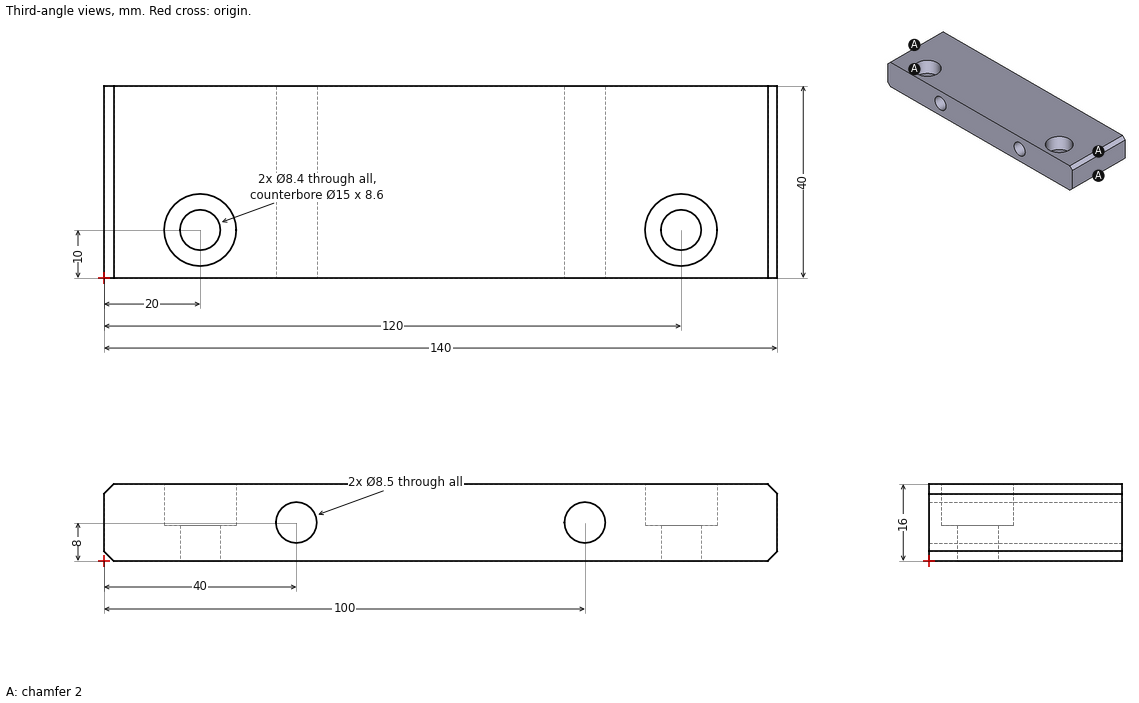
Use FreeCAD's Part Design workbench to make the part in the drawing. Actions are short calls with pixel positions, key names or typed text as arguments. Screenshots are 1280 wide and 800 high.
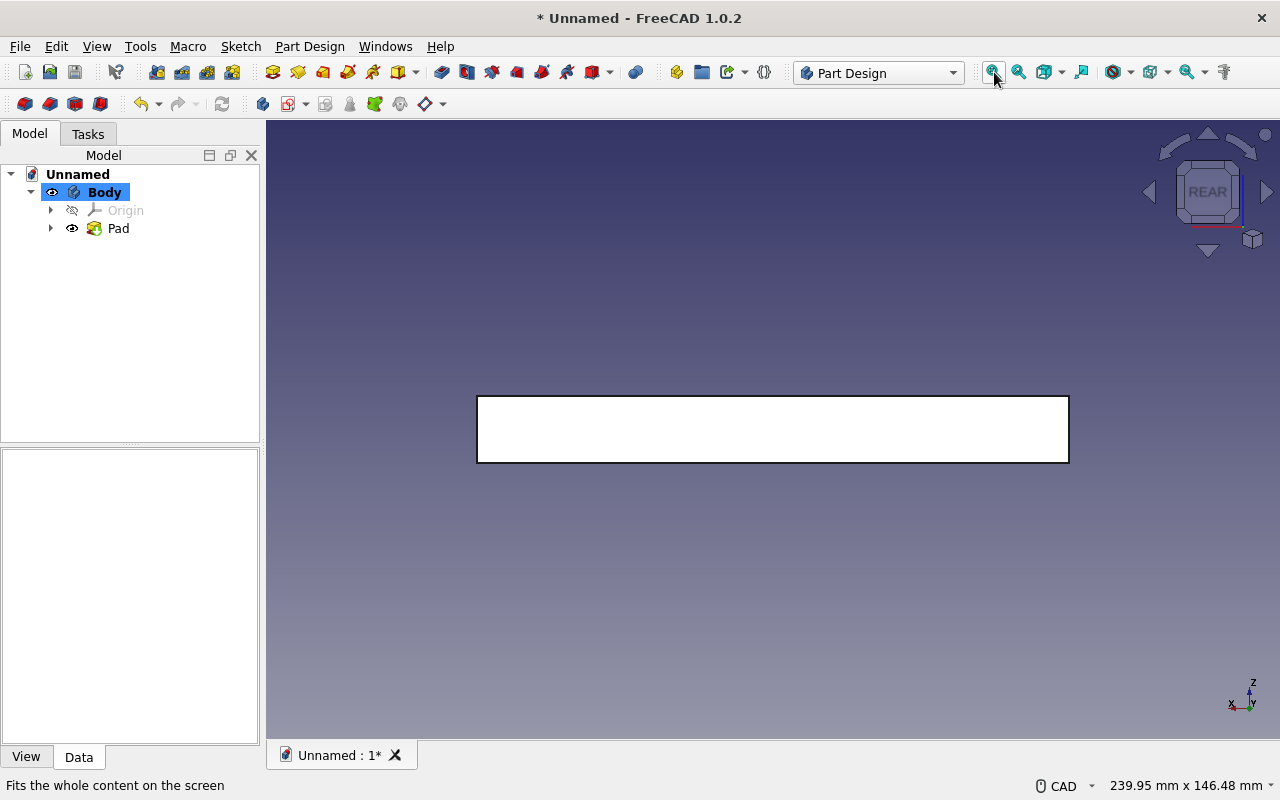
click(519, 428)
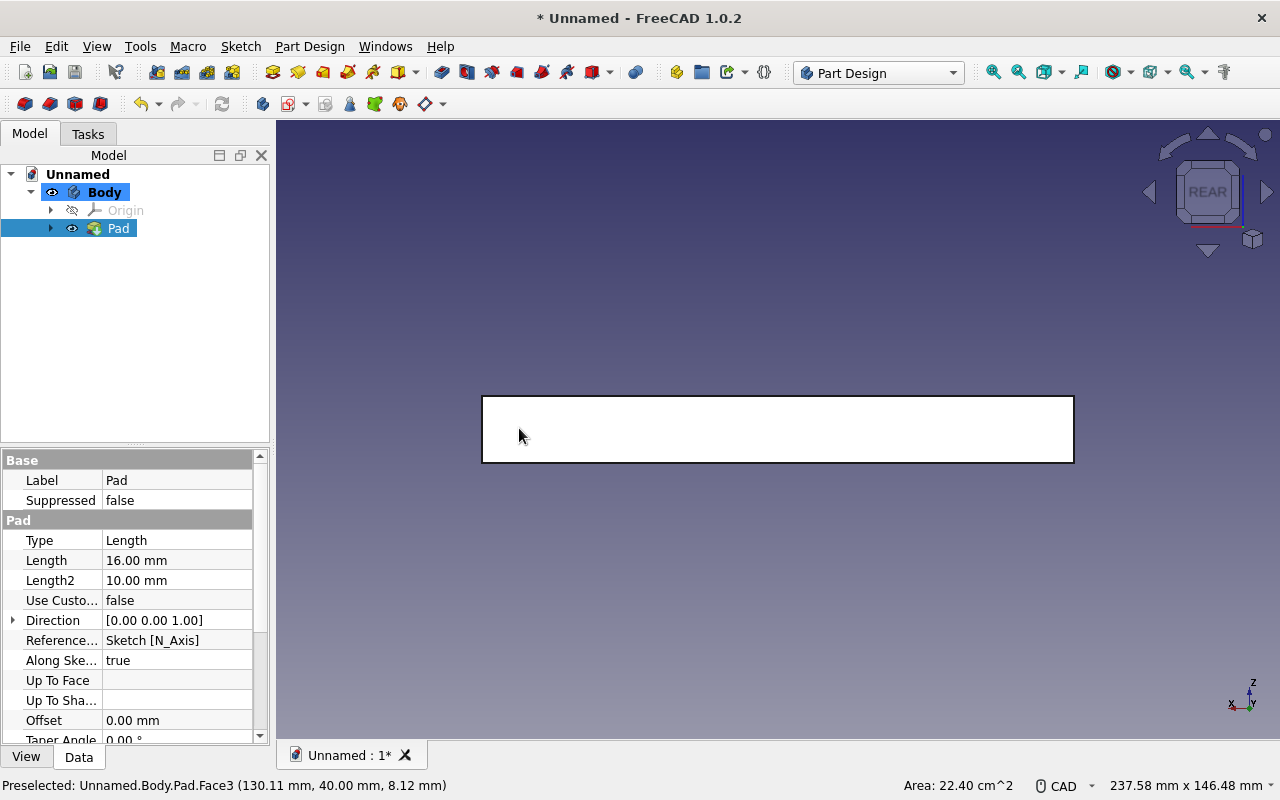
click(288, 104)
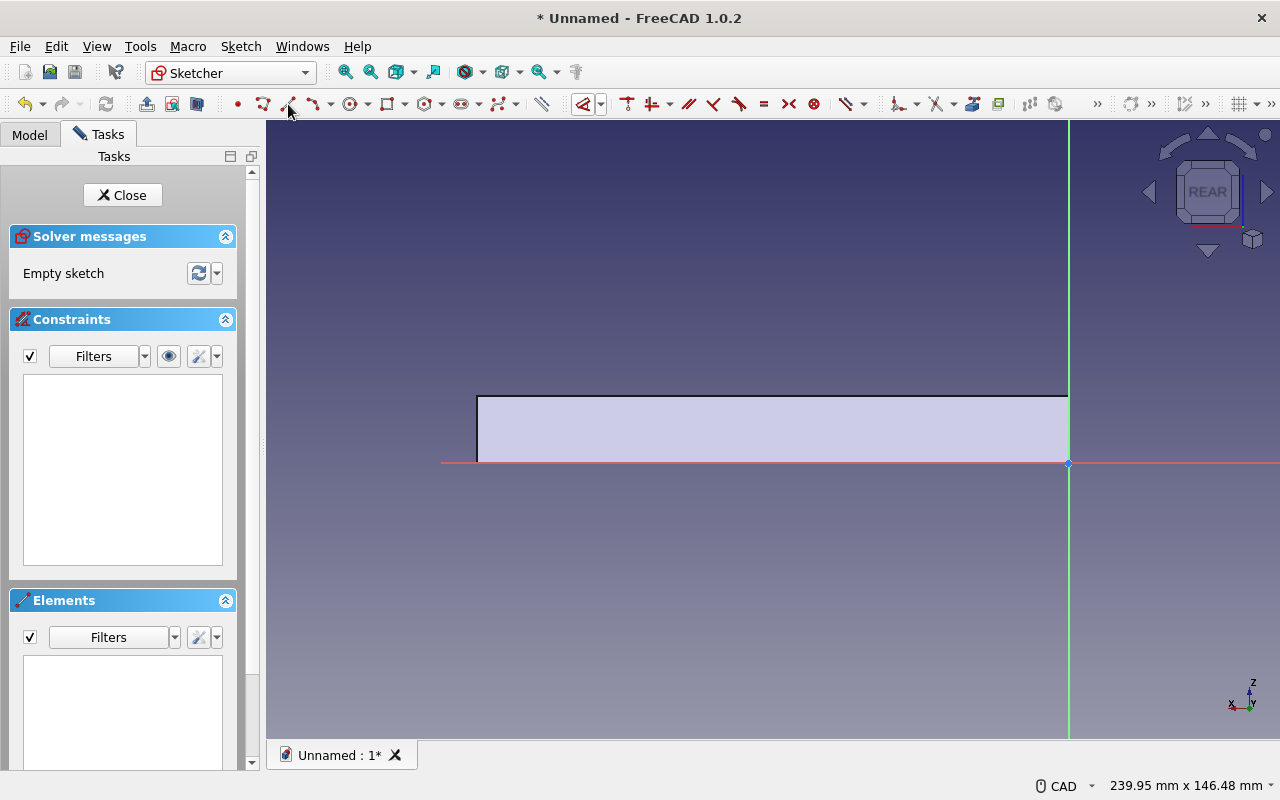
click(350, 104)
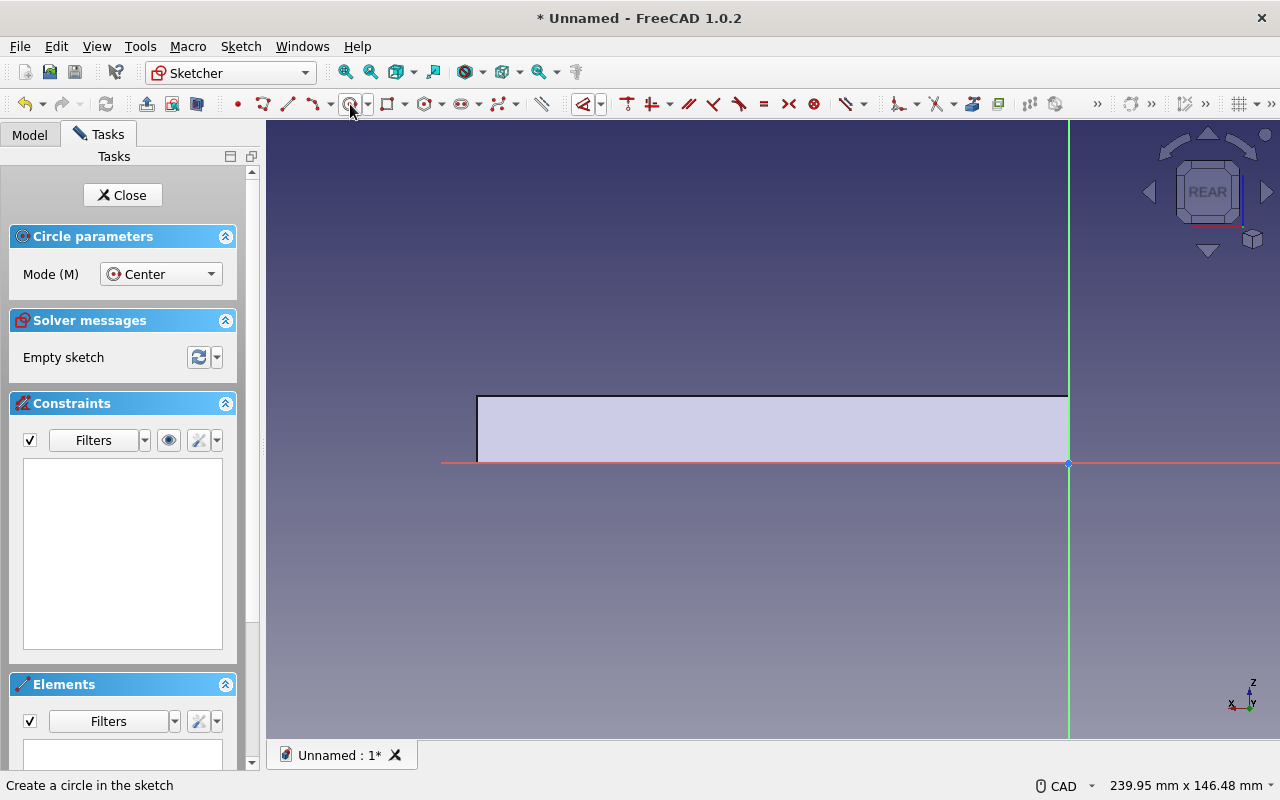
scroll(900, 429, up, 2)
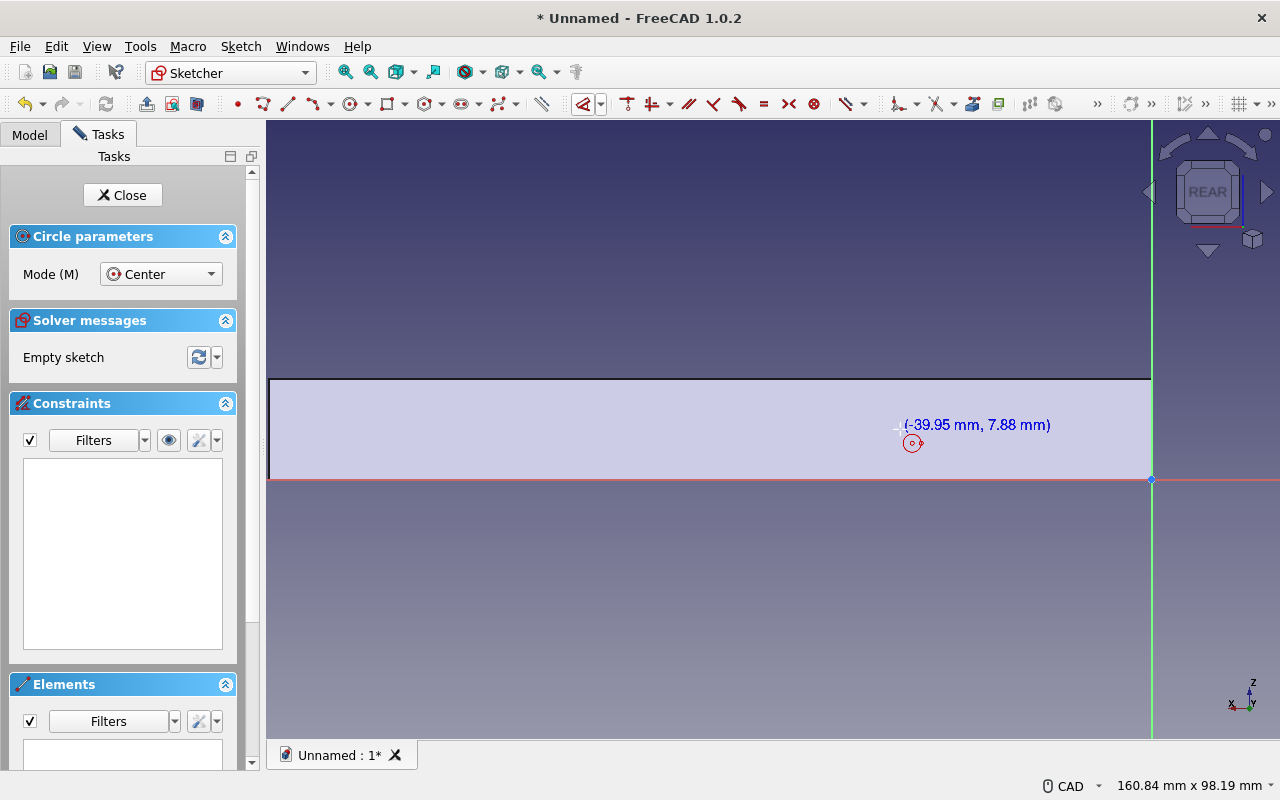
click(899, 429)
click(918, 411)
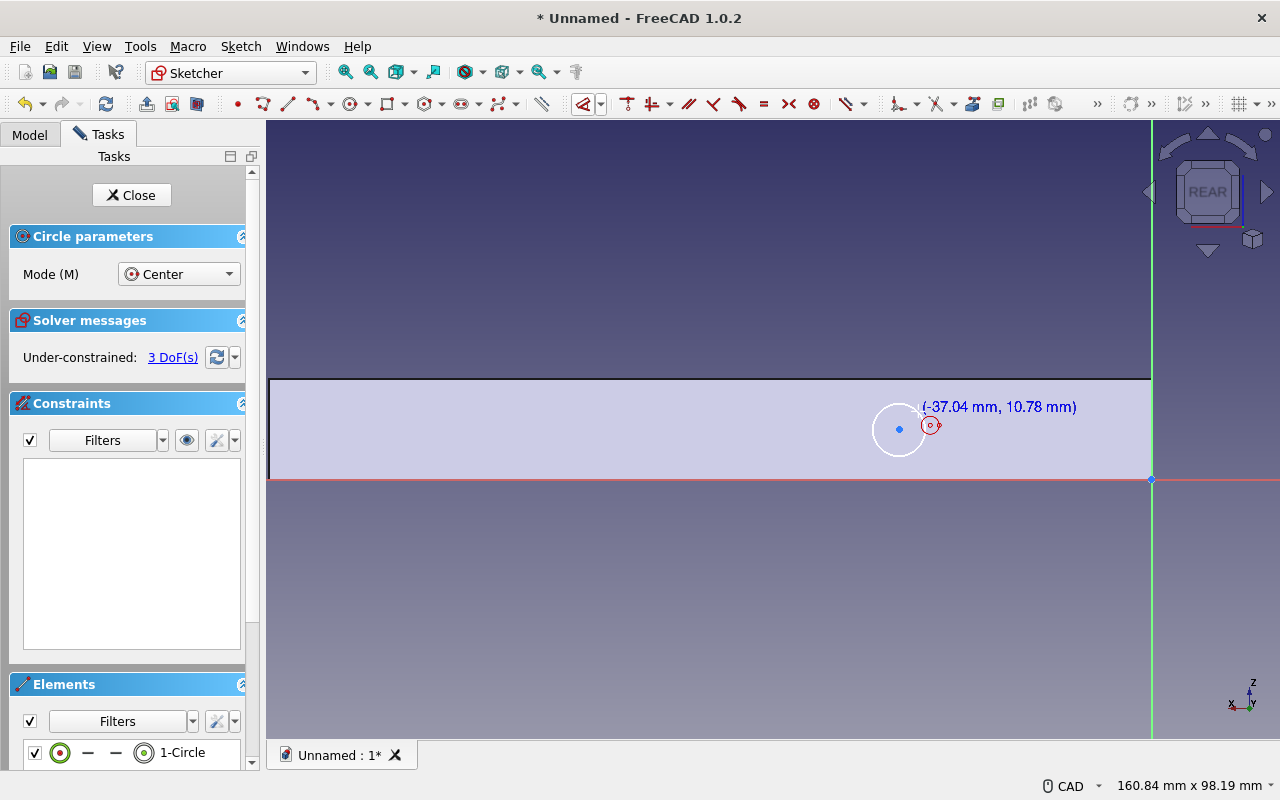
click(521, 429)
click(540, 411)
key(Escape)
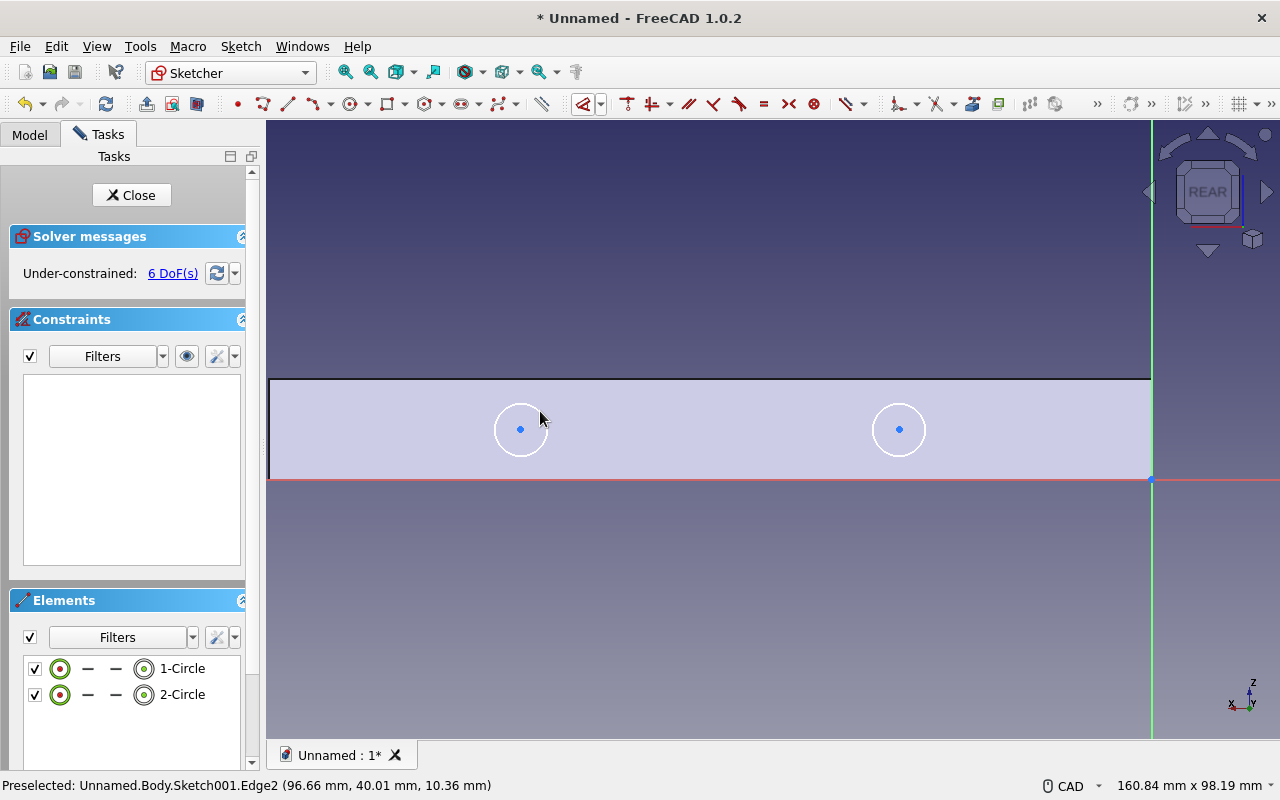
click(917, 411)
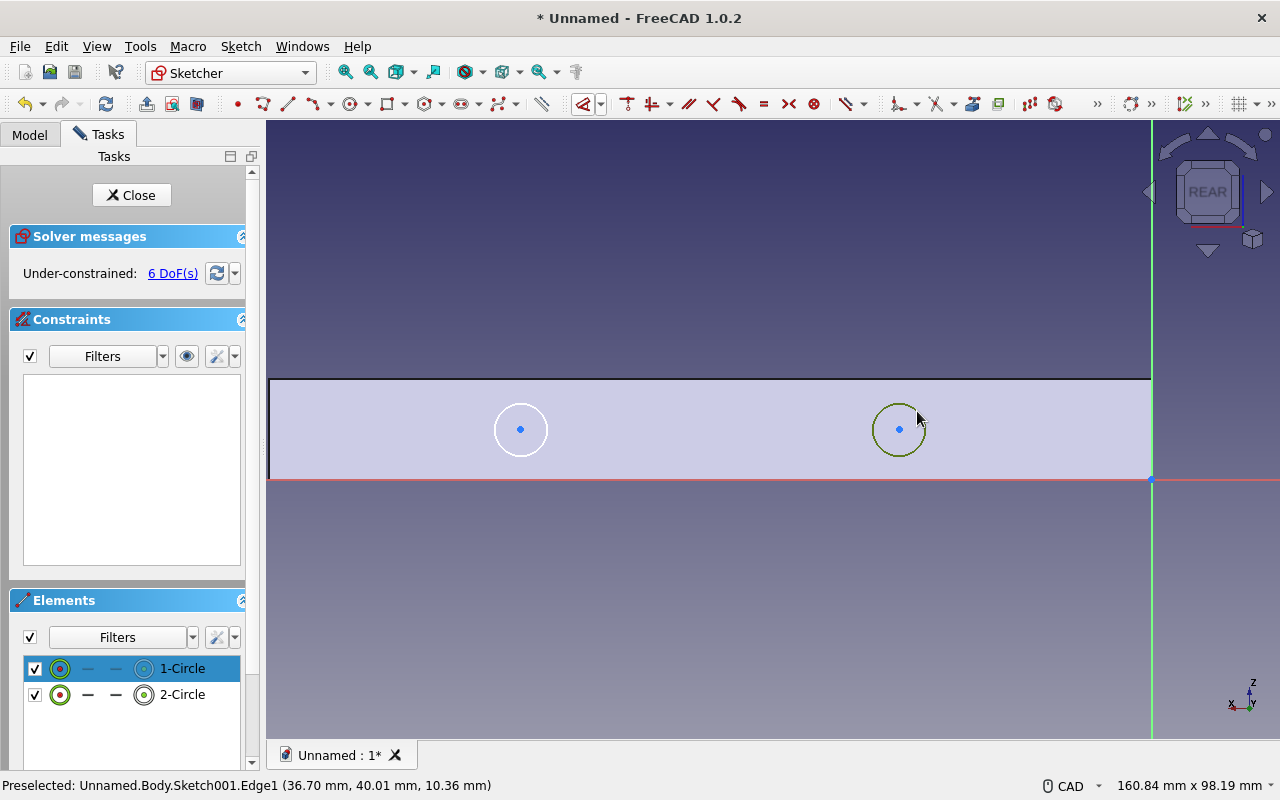
click(539, 411)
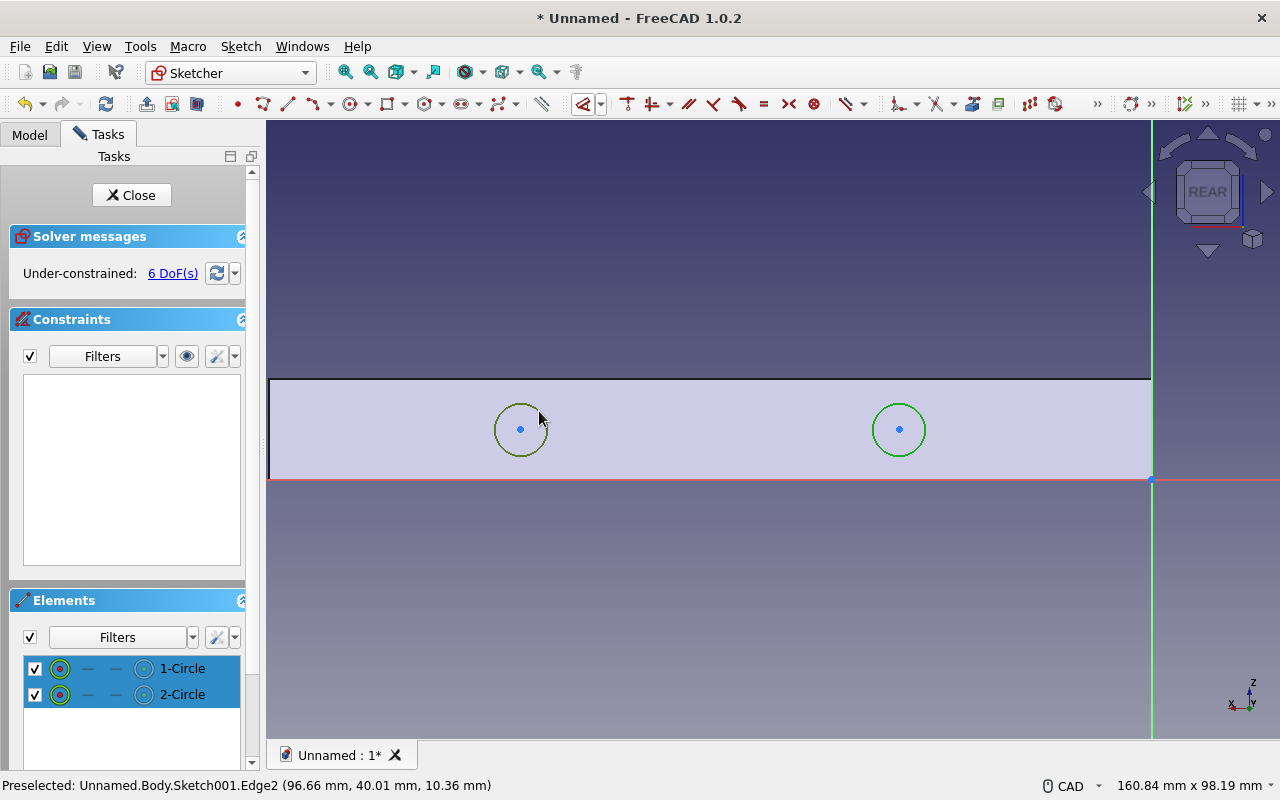
click(764, 104)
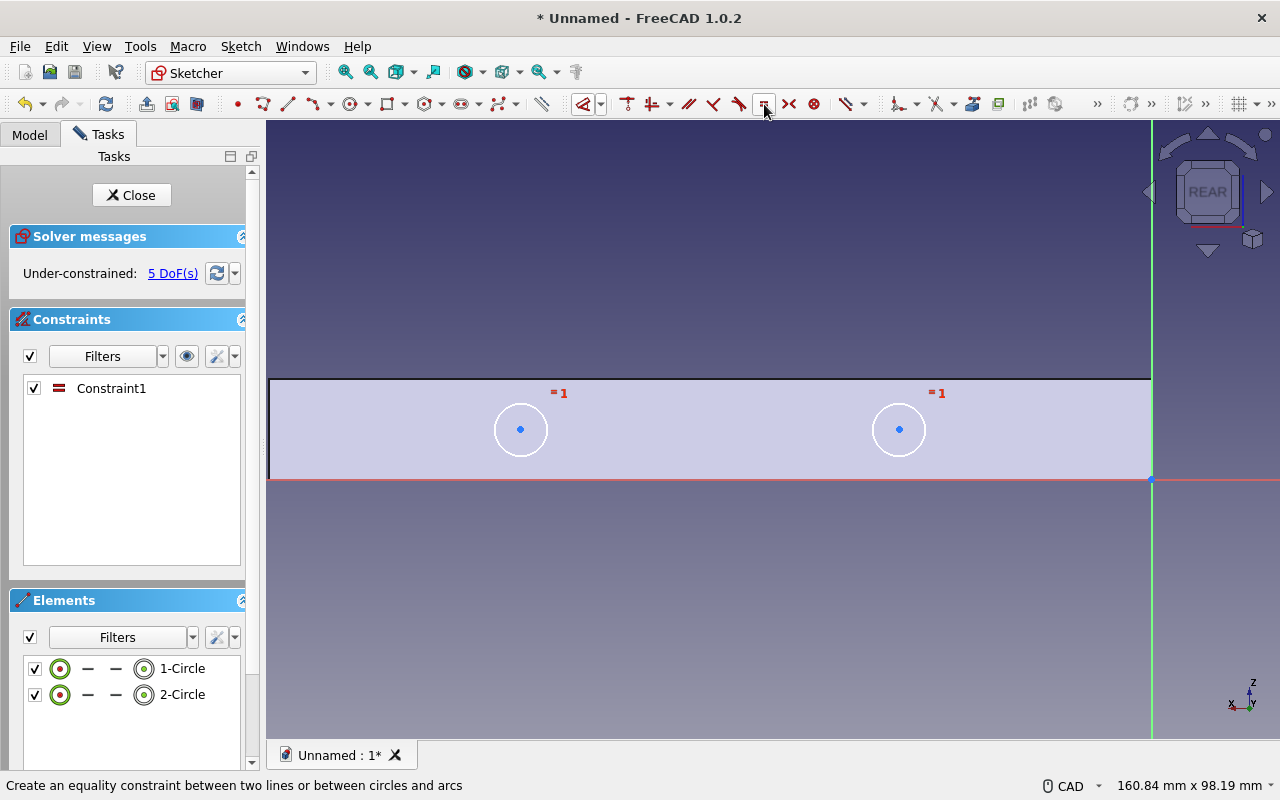
click(917, 411)